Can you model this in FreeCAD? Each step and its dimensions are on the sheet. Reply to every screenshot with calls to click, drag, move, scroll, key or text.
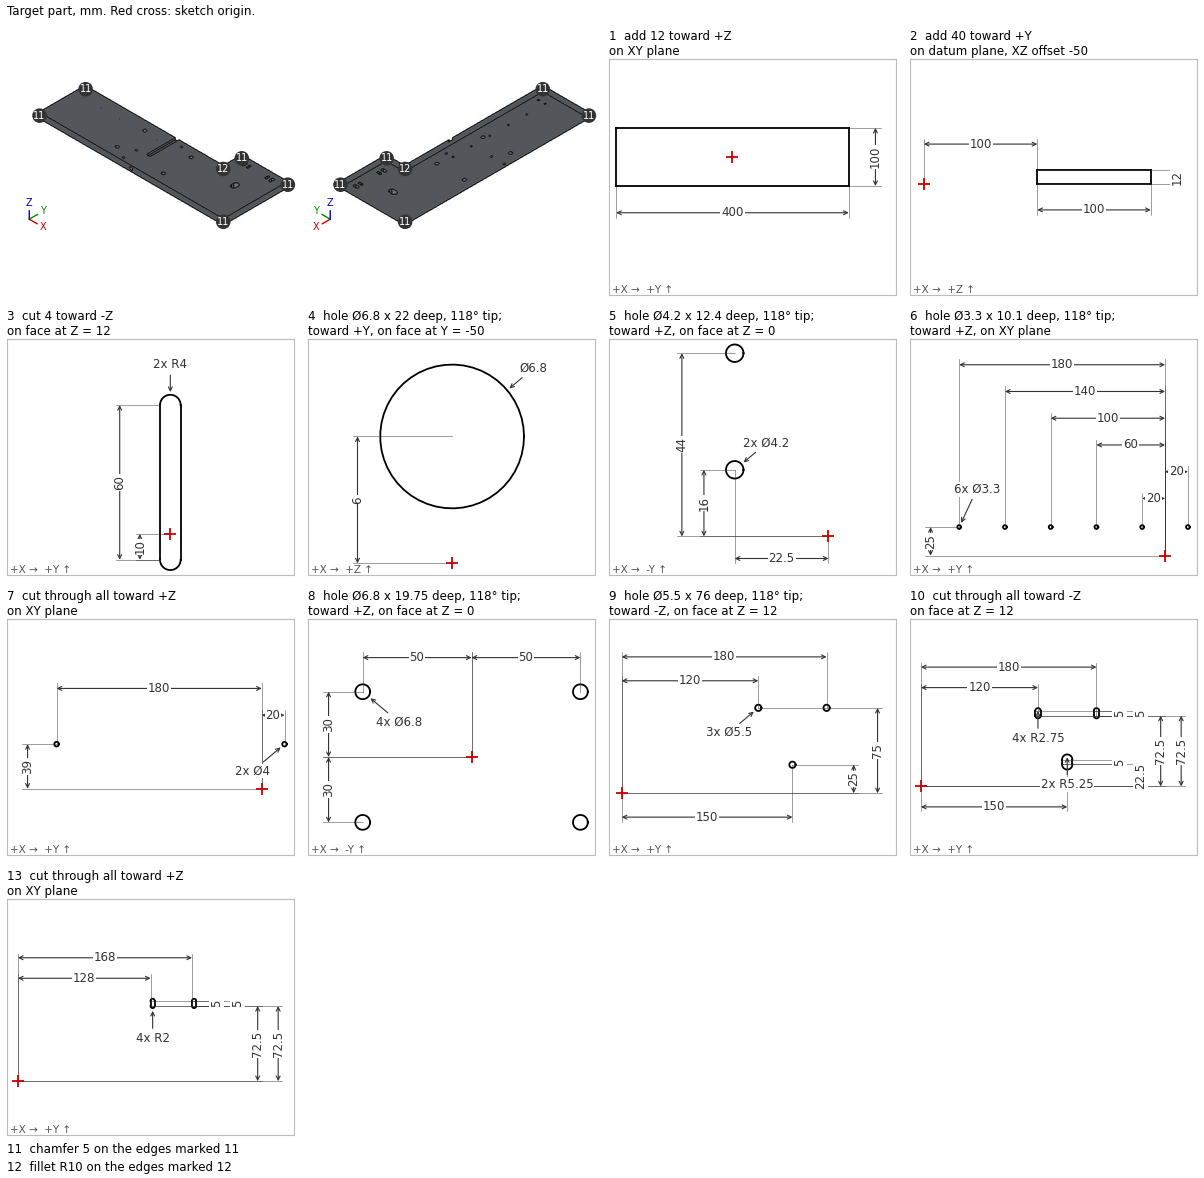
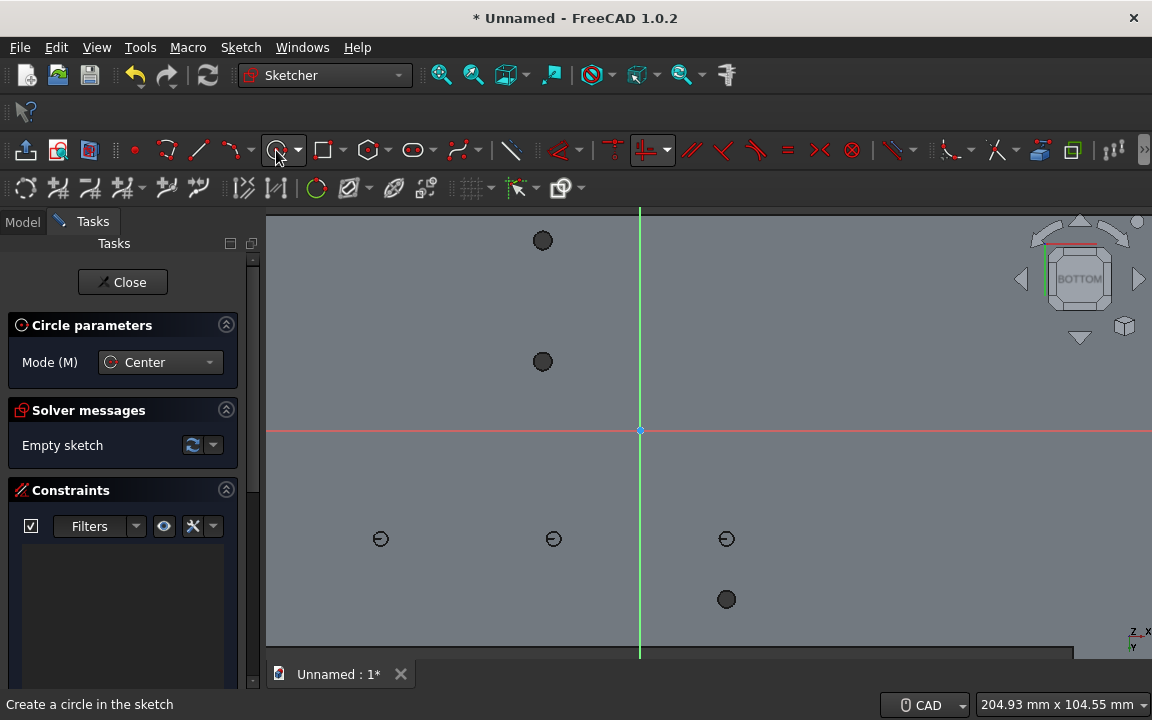
scroll(424, 301, up, 3)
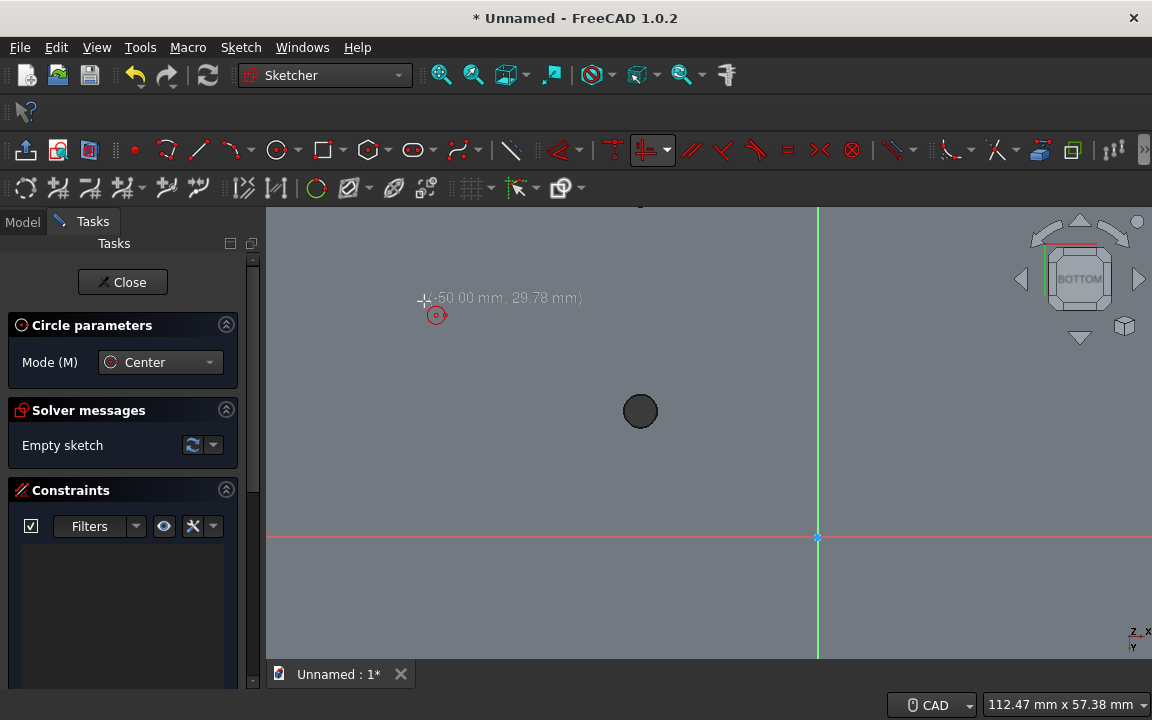
click(424, 301)
move(443, 282)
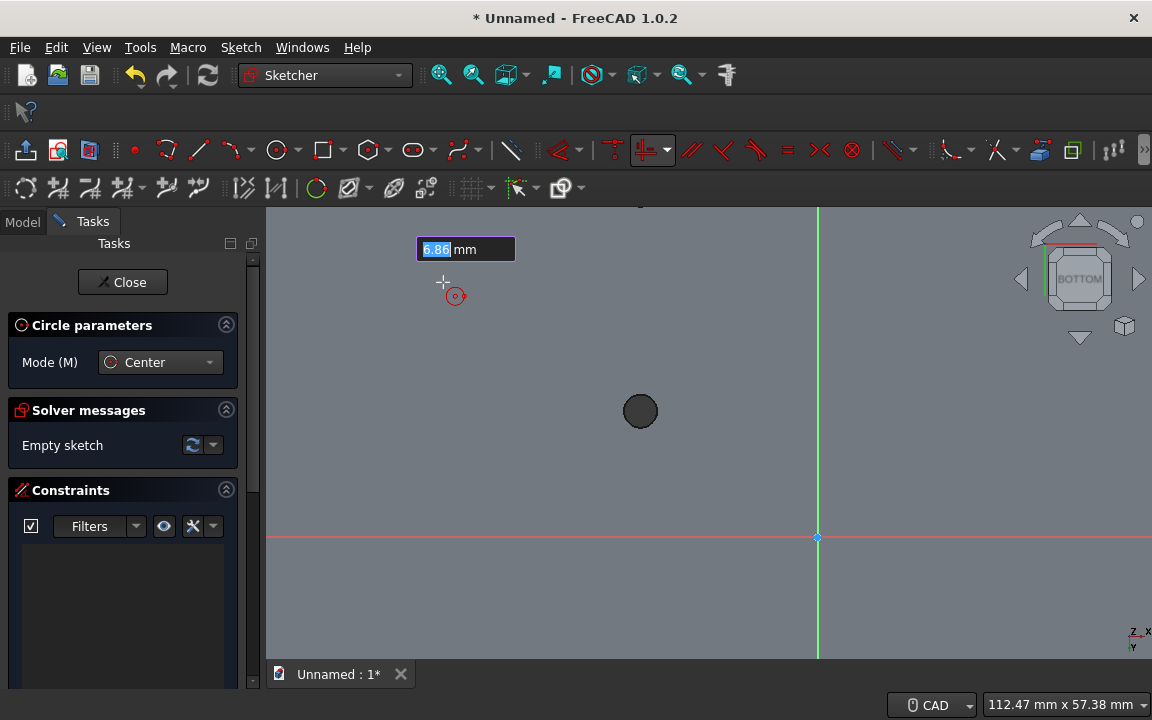
text(6.8)
key(Return)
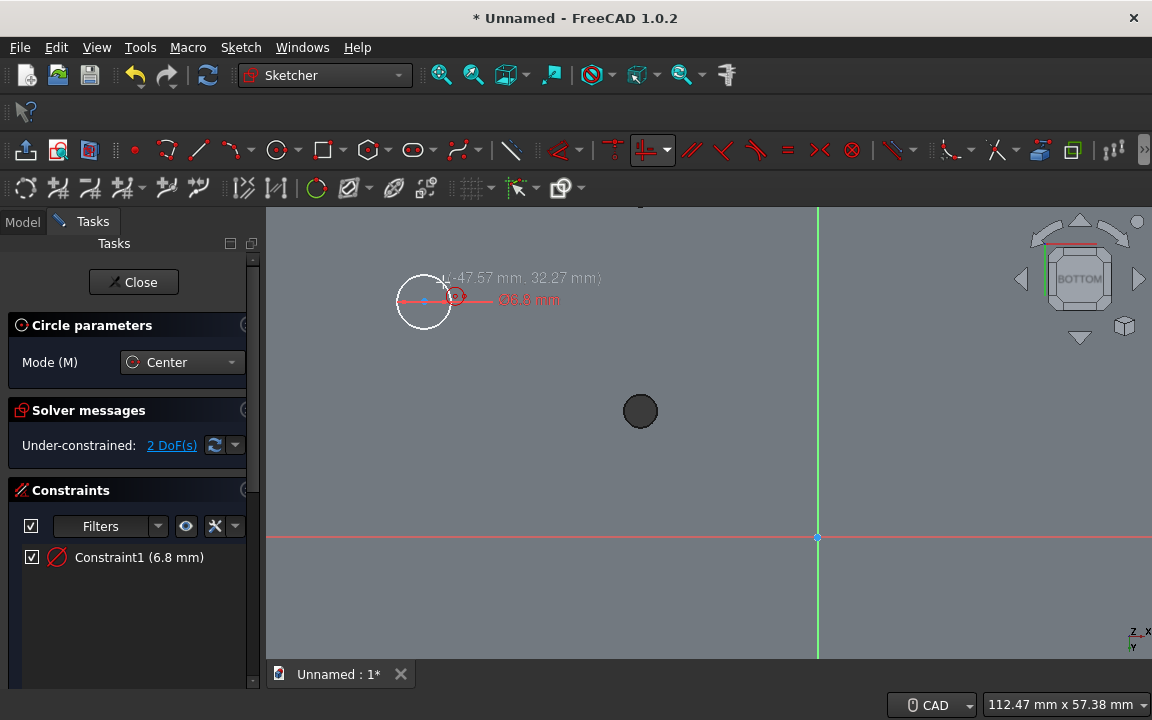
scroll(425, 306, down, 3)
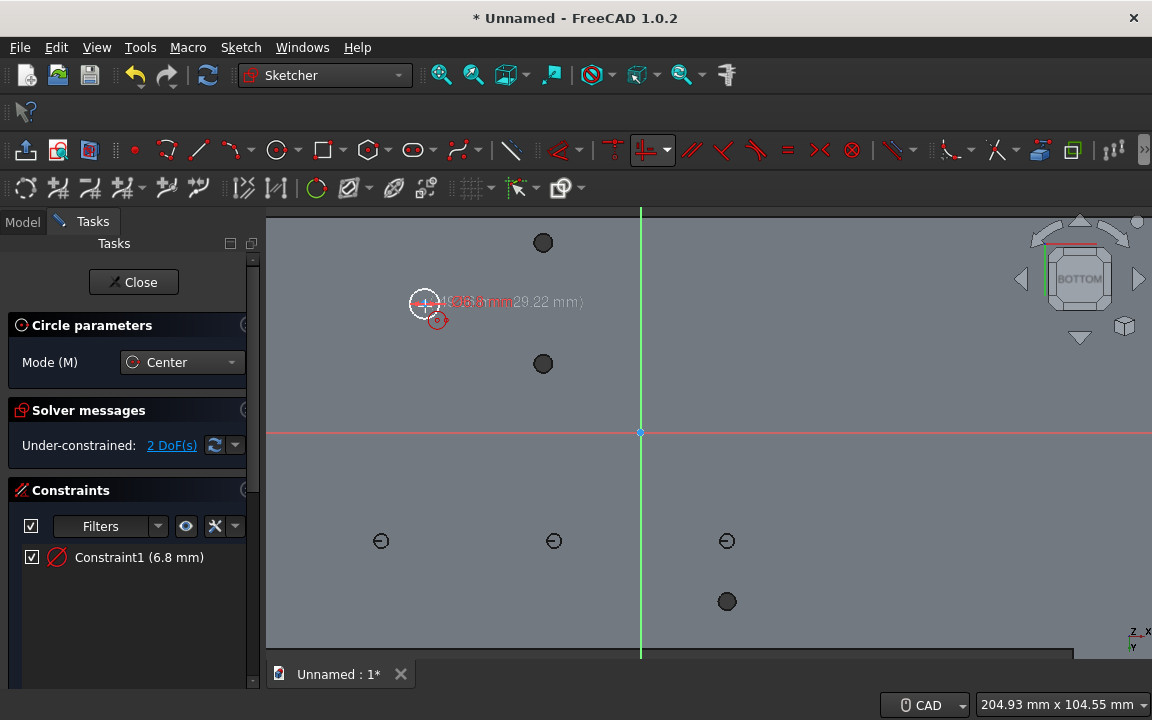
scroll(424, 563, up, 3)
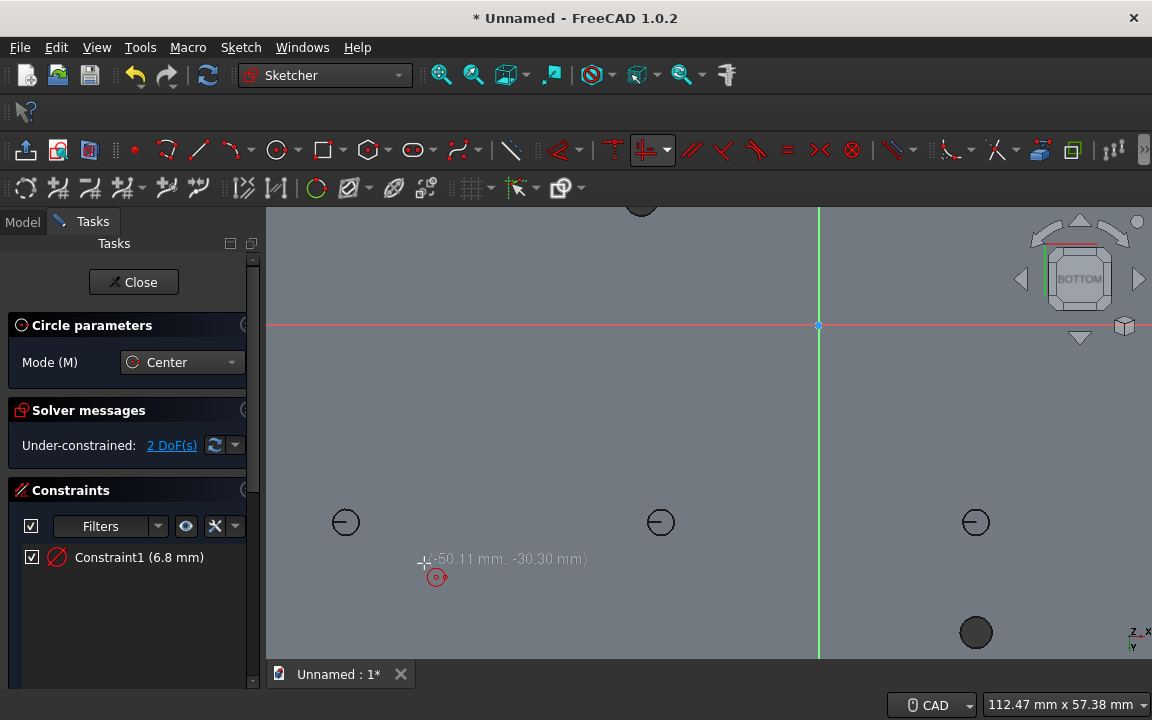
click(425, 562)
move(444, 543)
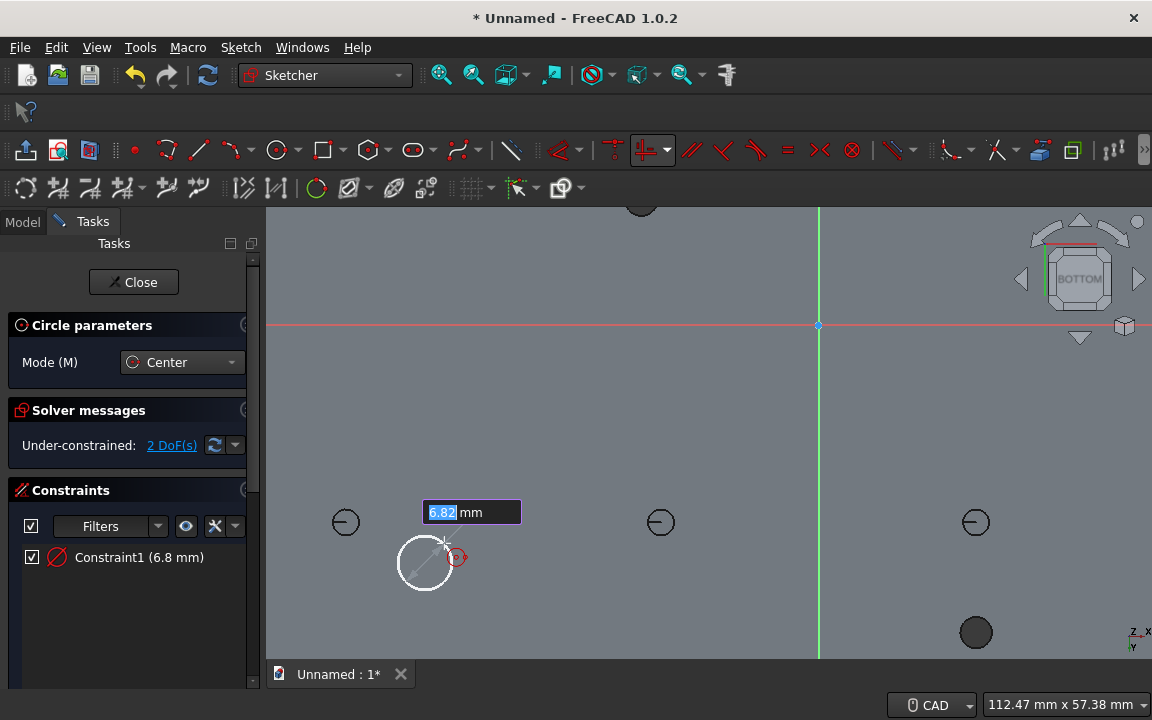
text(6.8)
key(Return)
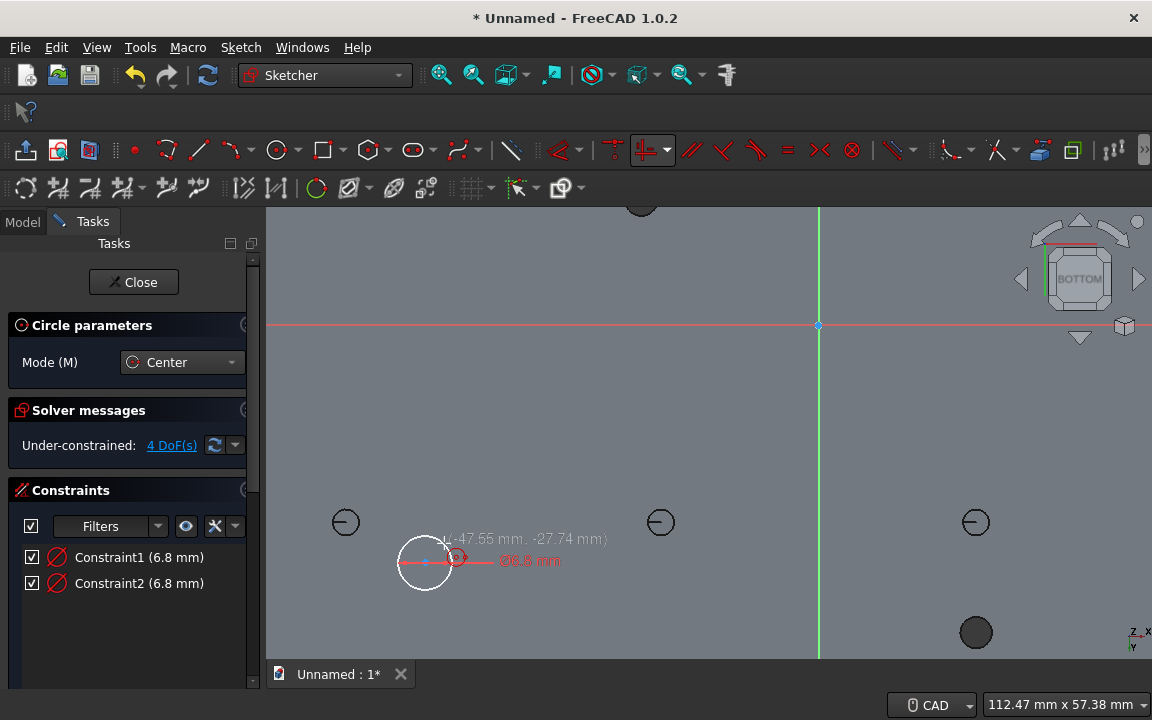
scroll(424, 564, down, 3)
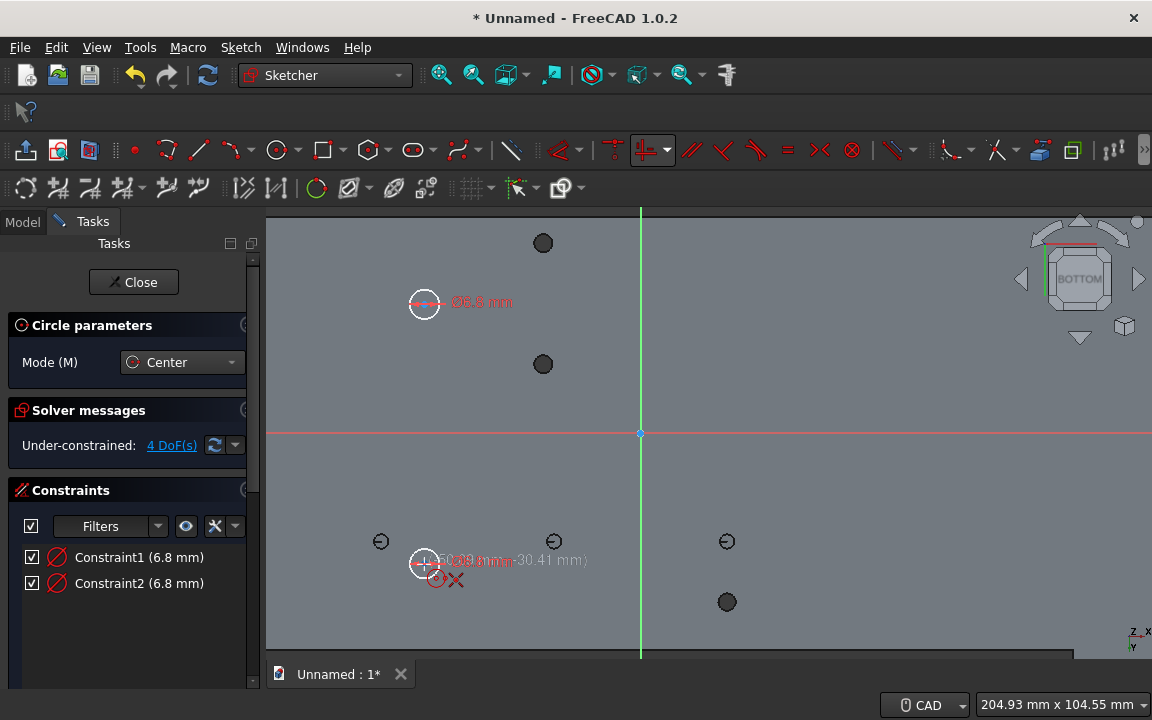
scroll(857, 304, up, 3)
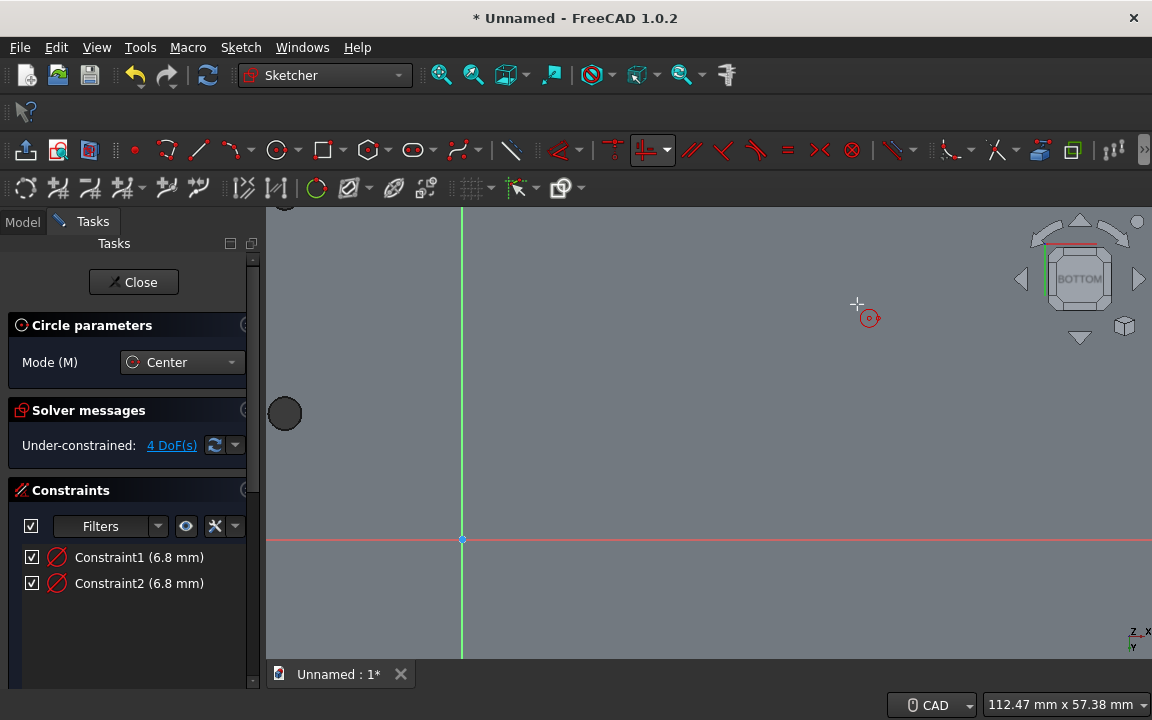
click(856, 303)
move(875, 284)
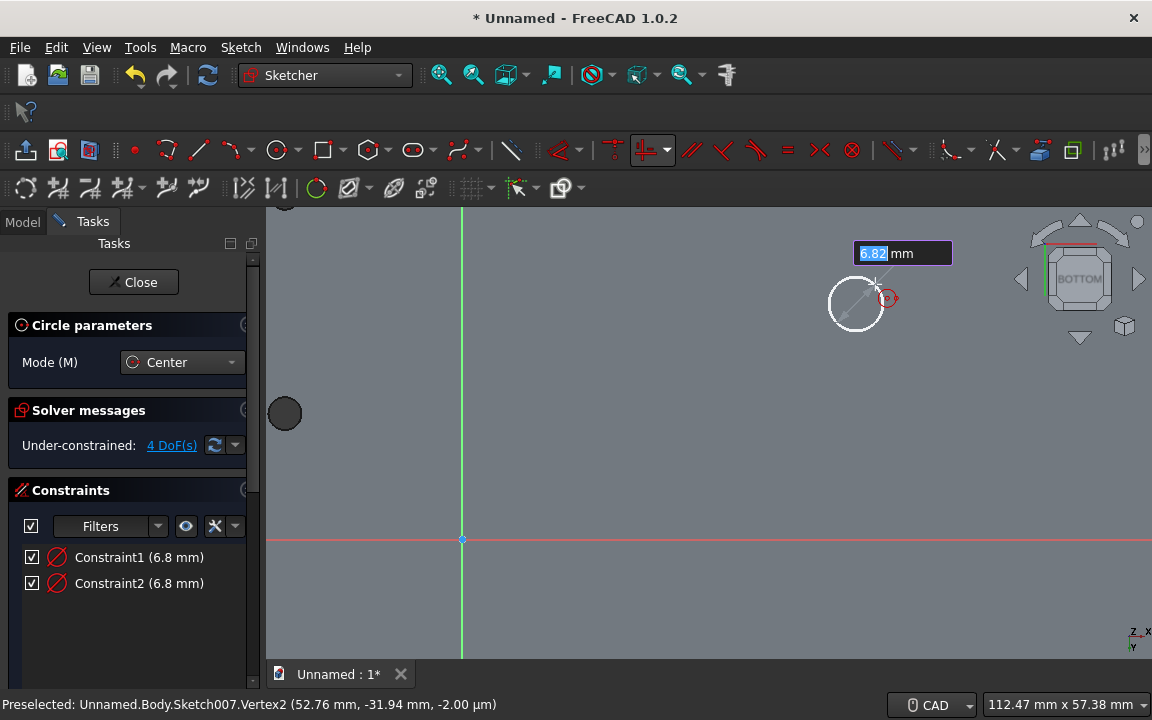
text(6.8)
key(Return)